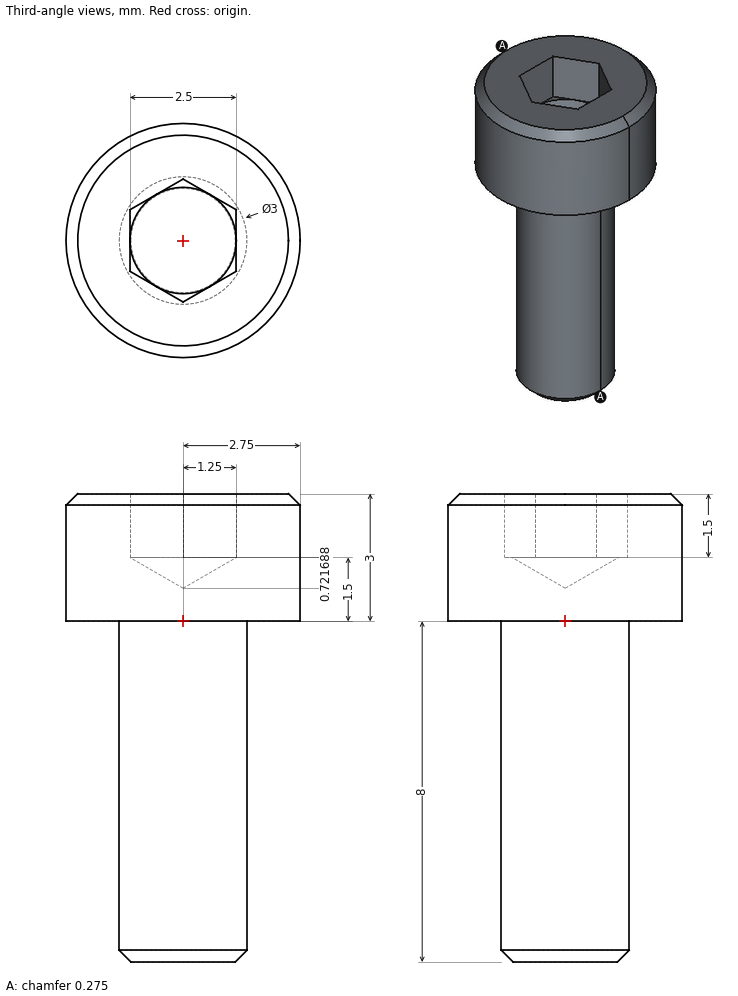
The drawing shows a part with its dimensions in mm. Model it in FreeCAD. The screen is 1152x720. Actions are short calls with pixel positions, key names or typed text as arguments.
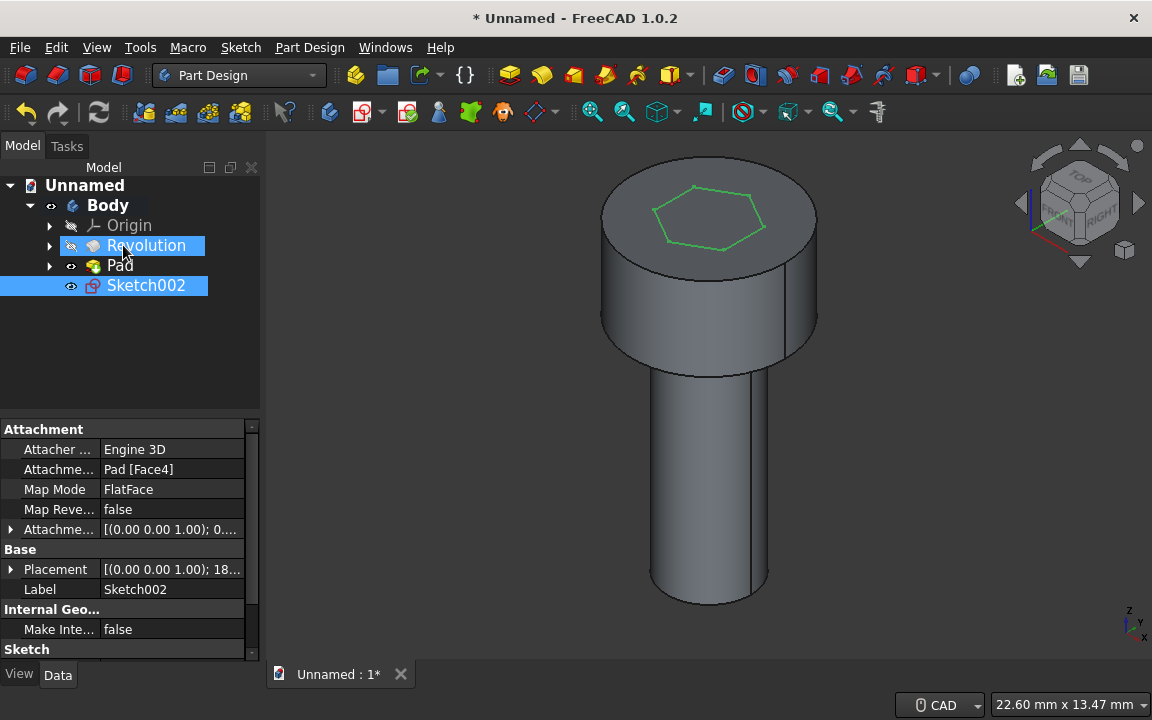
click(724, 76)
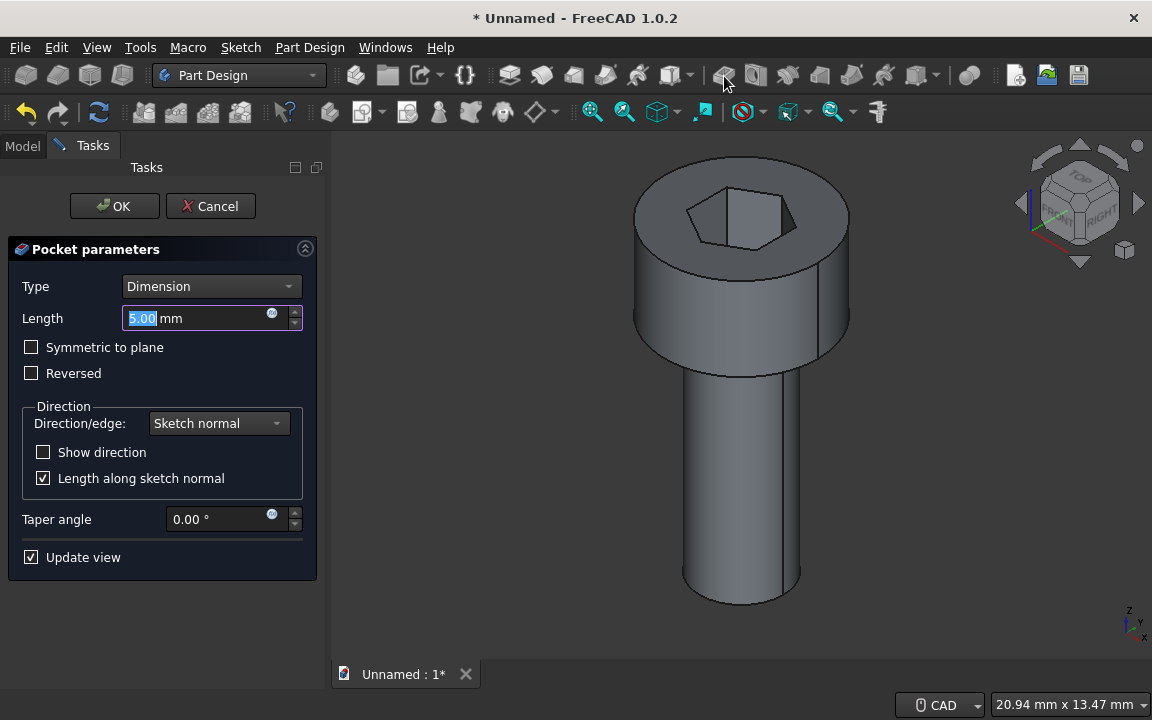
text(1.5)
key(Tab)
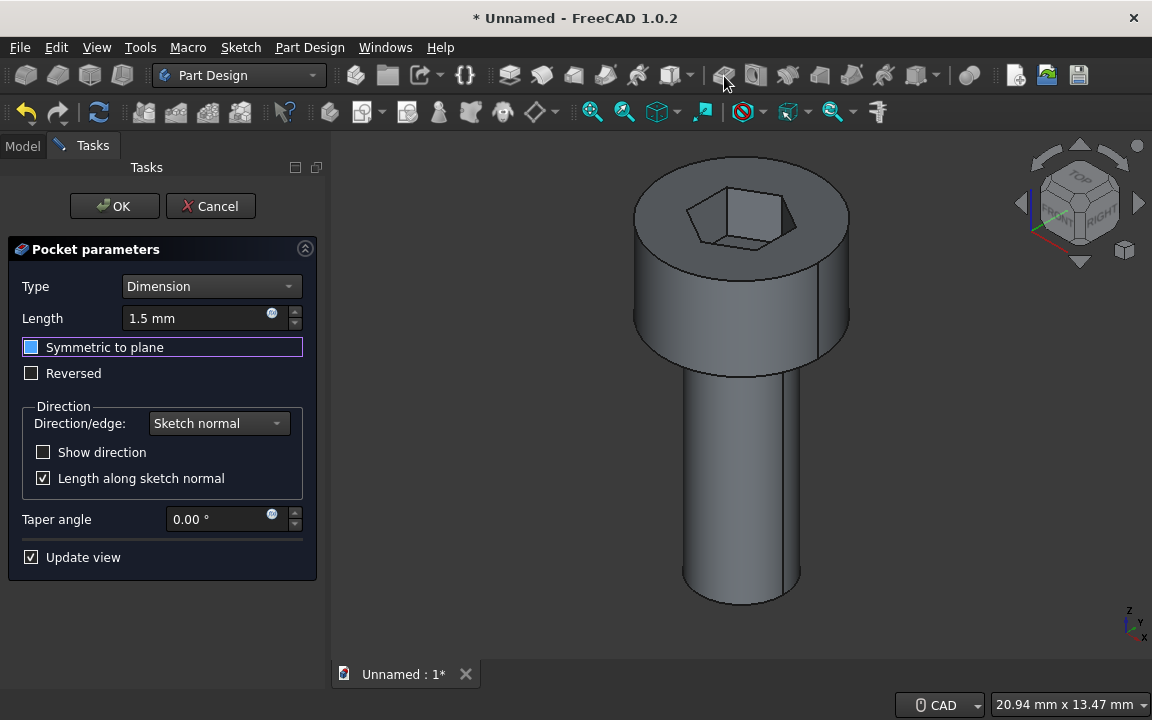
click(115, 206)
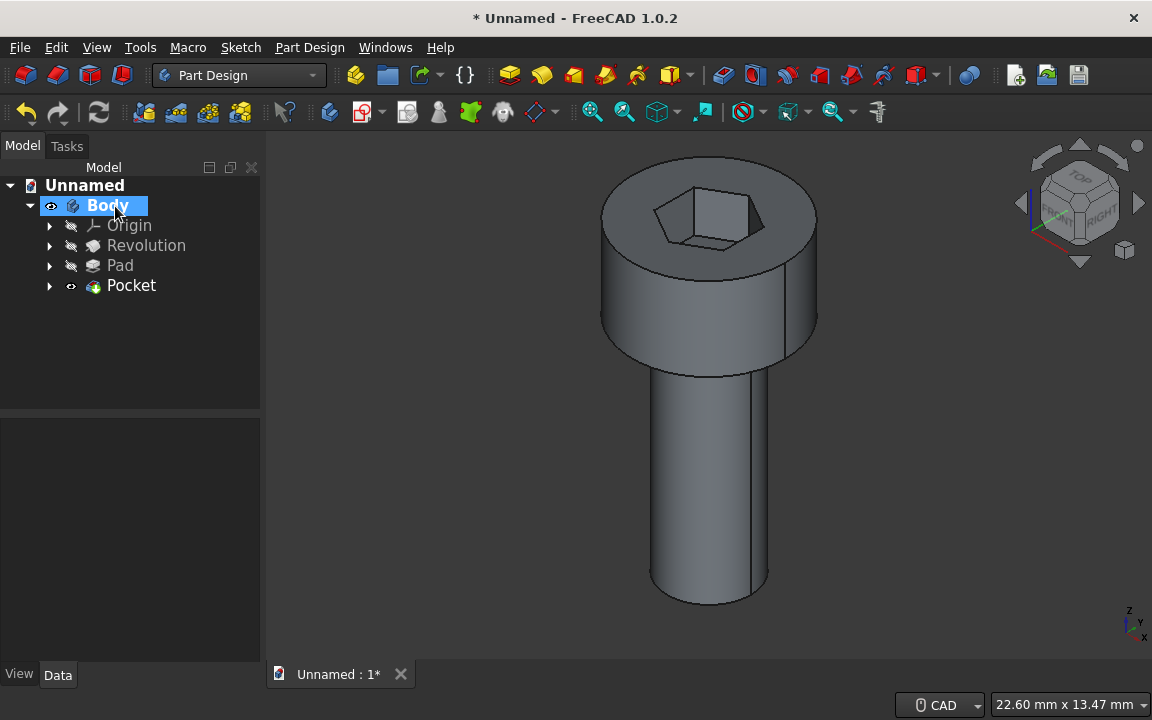
click(594, 112)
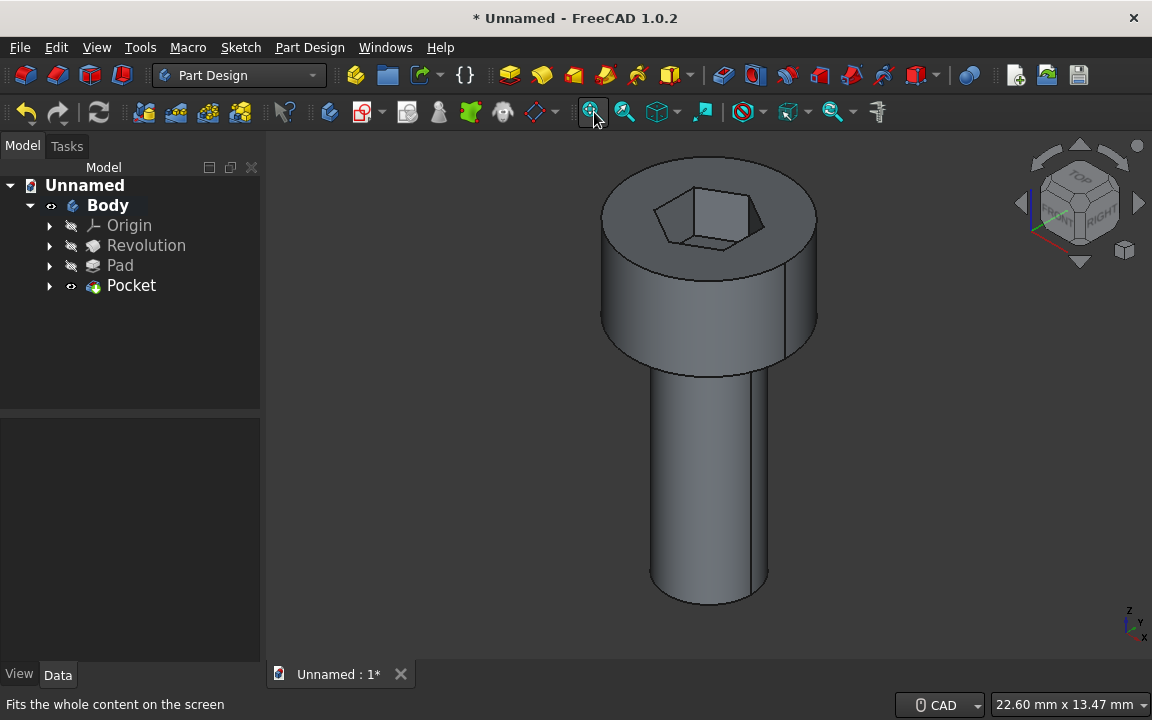
click(362, 112)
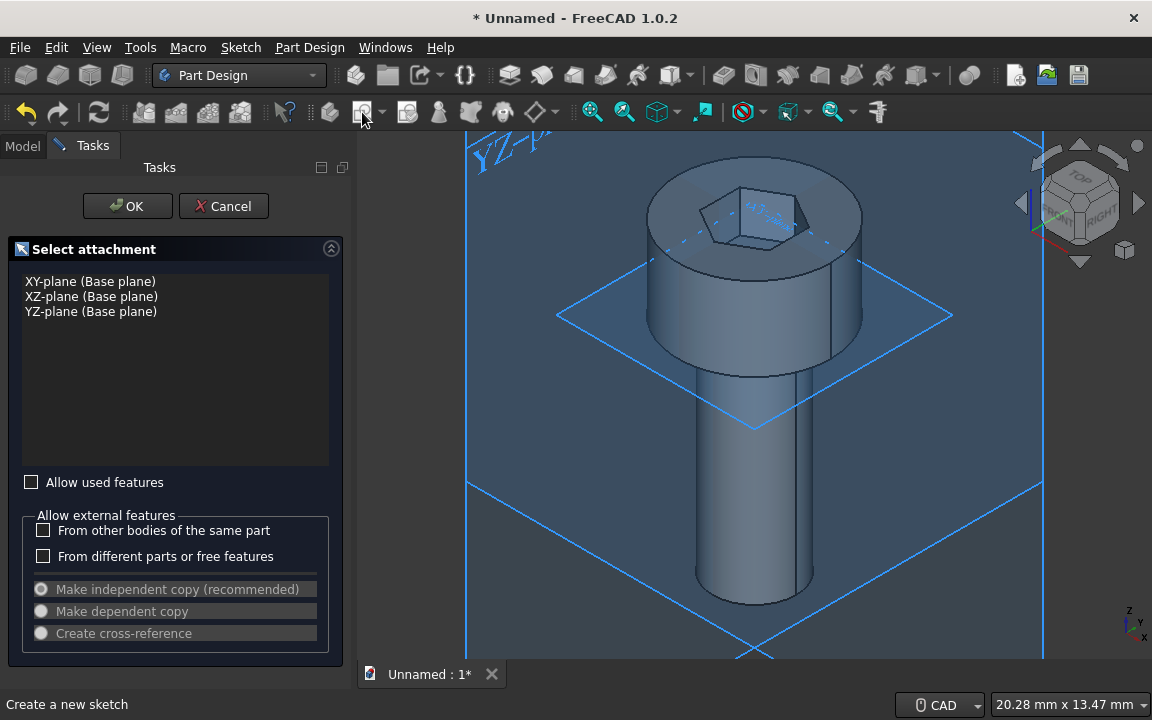
click(82, 296)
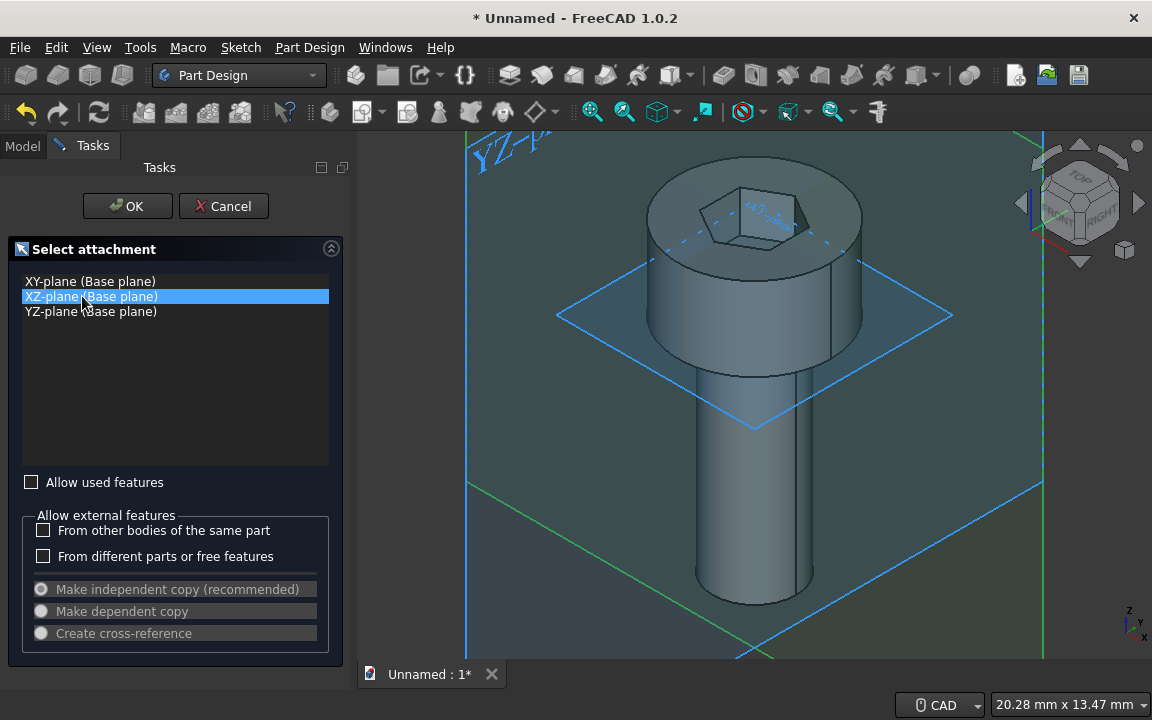
click(128, 206)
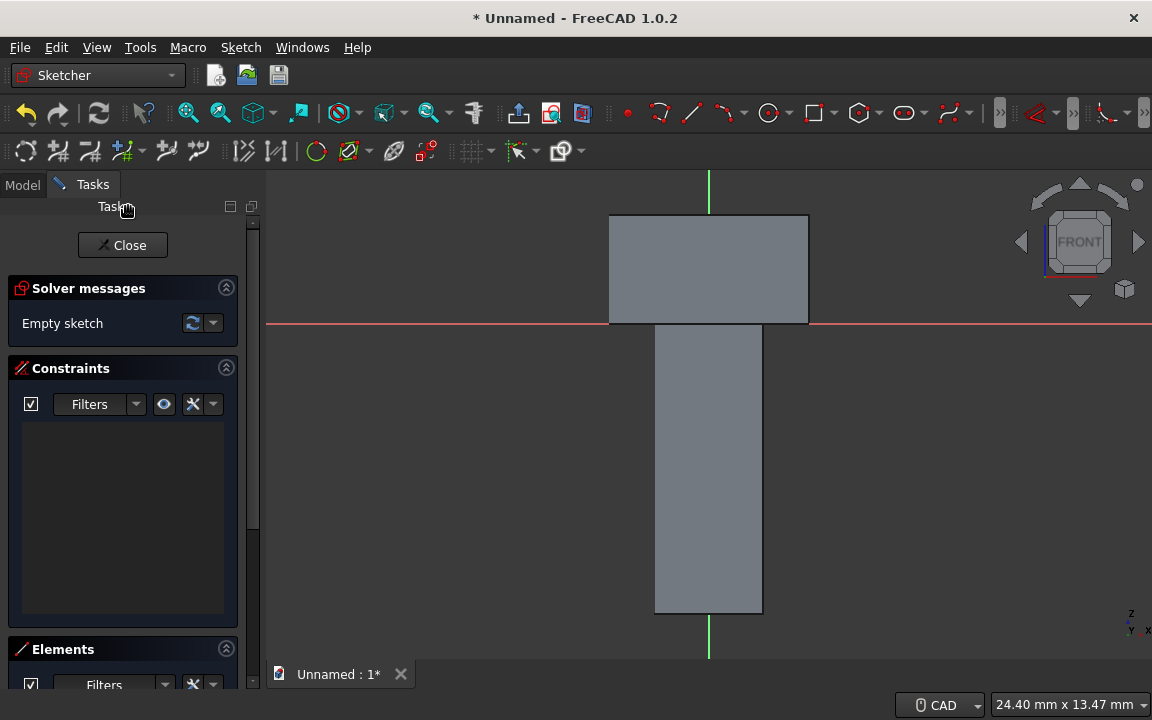
click(584, 114)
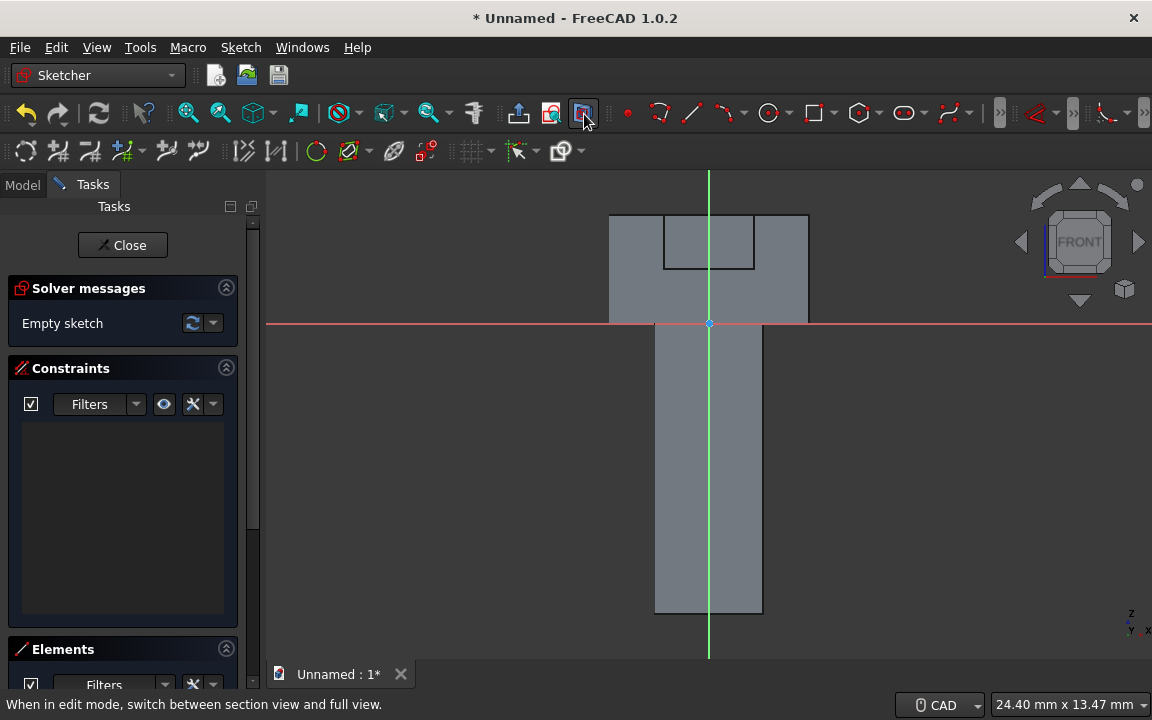
scroll(750, 273, up, 9)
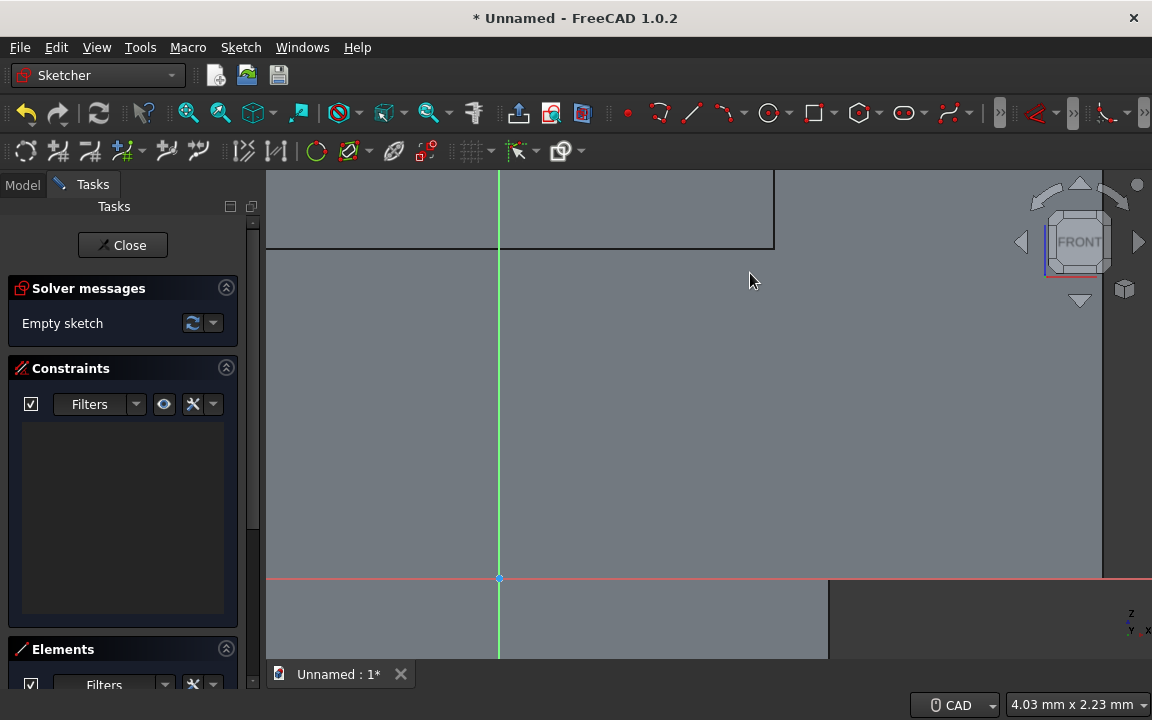
click(660, 114)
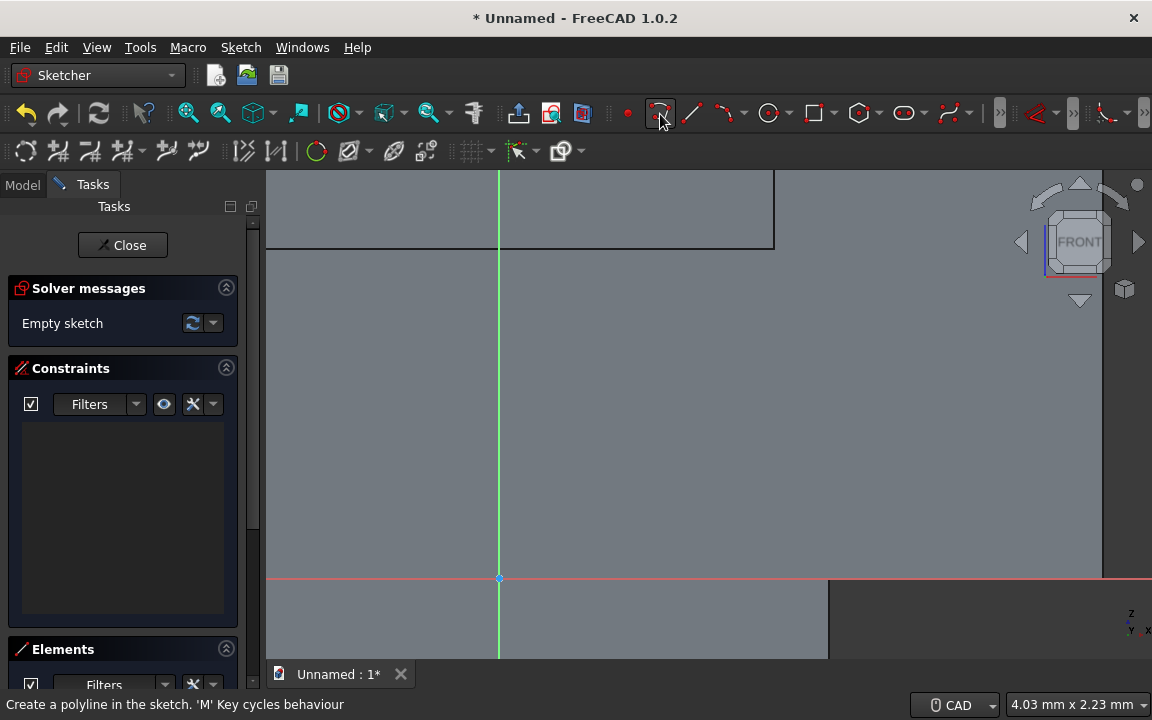
click(499, 408)
click(774, 249)
click(508, 249)
click(499, 409)
key(Escape)
key(Escape)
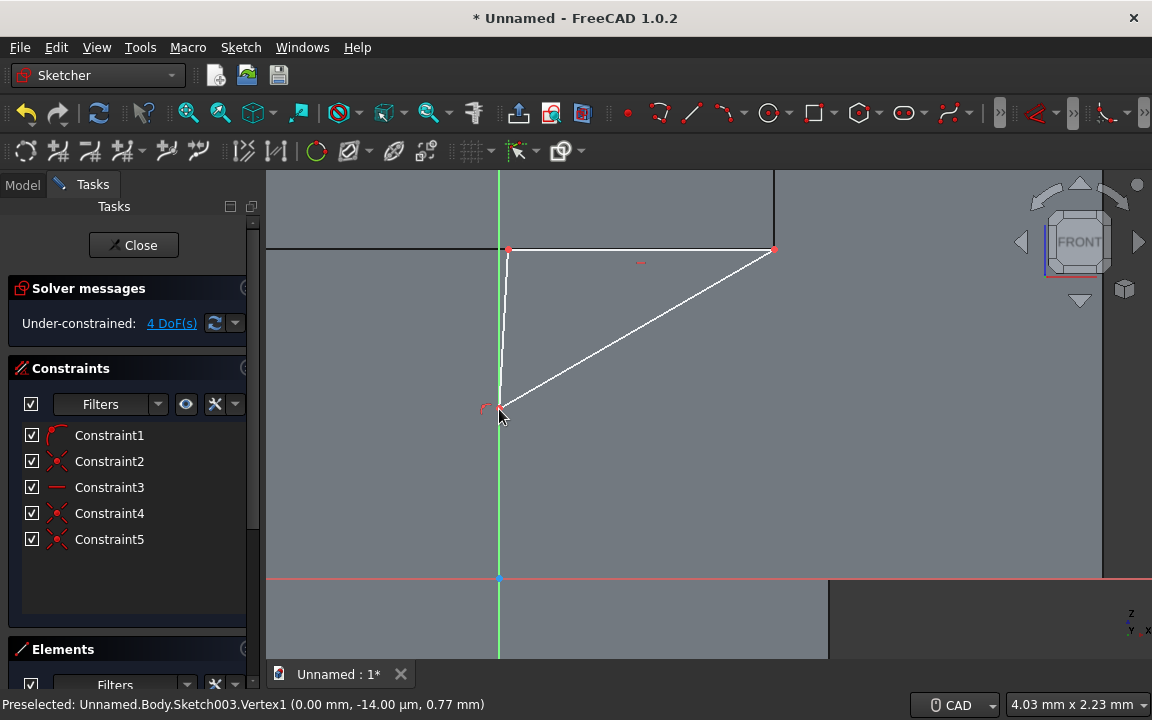
click(502, 361)